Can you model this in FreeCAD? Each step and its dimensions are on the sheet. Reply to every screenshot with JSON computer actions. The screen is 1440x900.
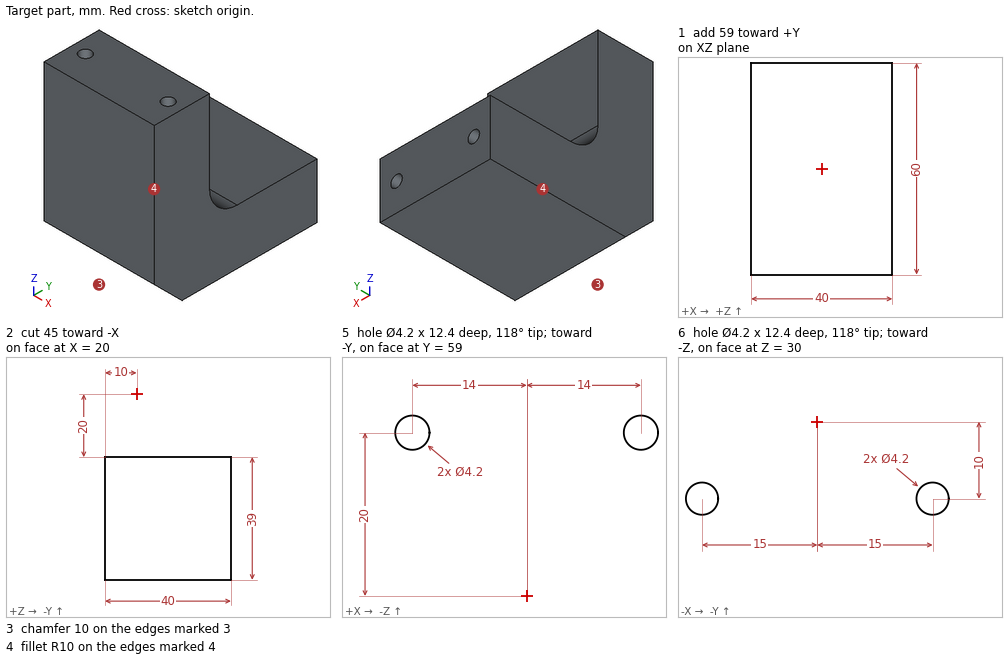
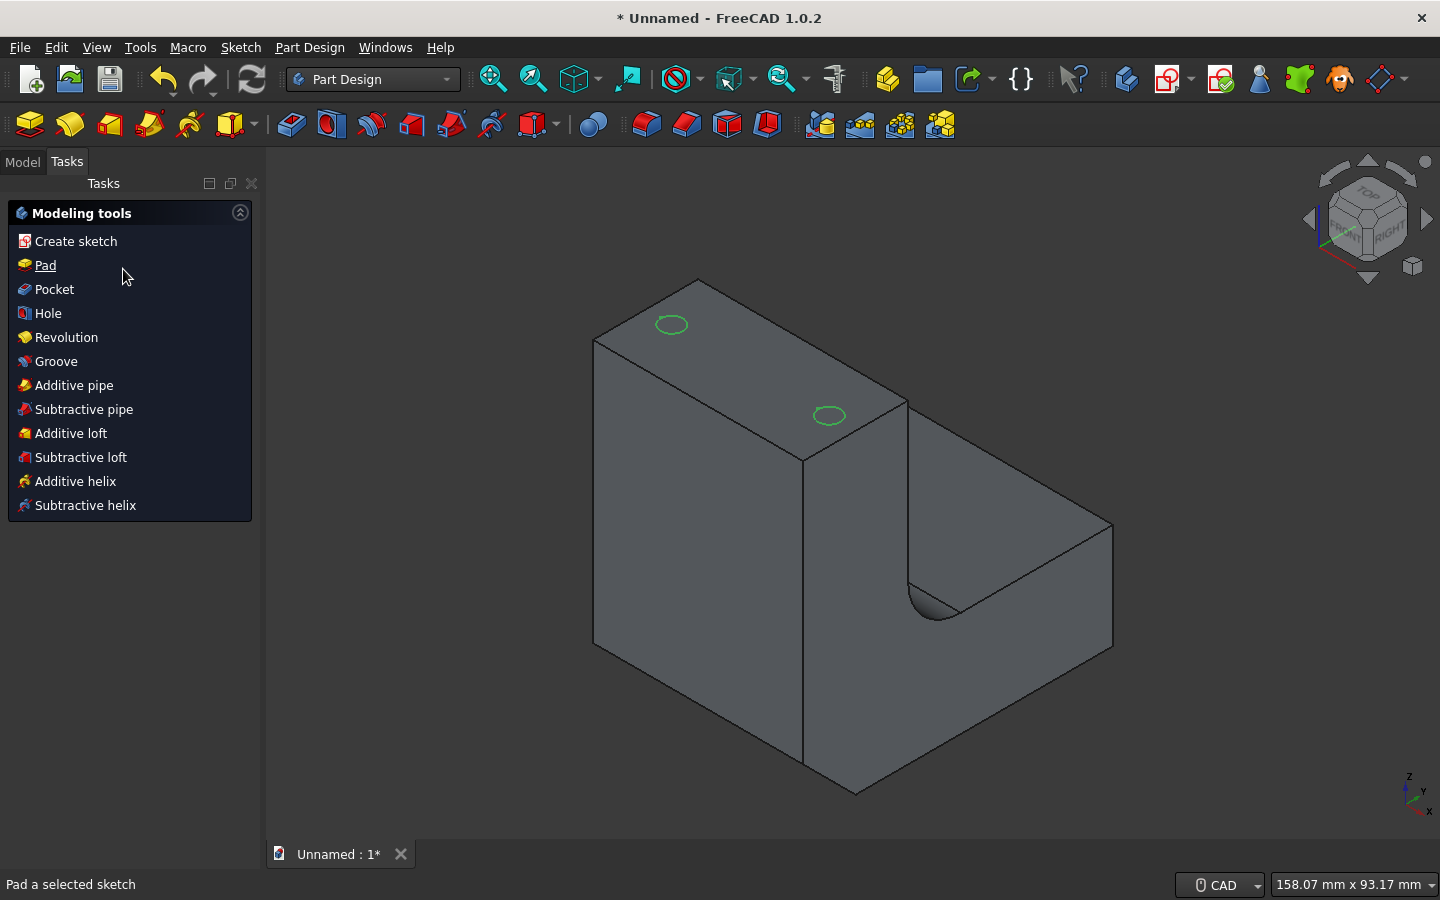
{"action": "left_click", "coordinate": [332, 124]}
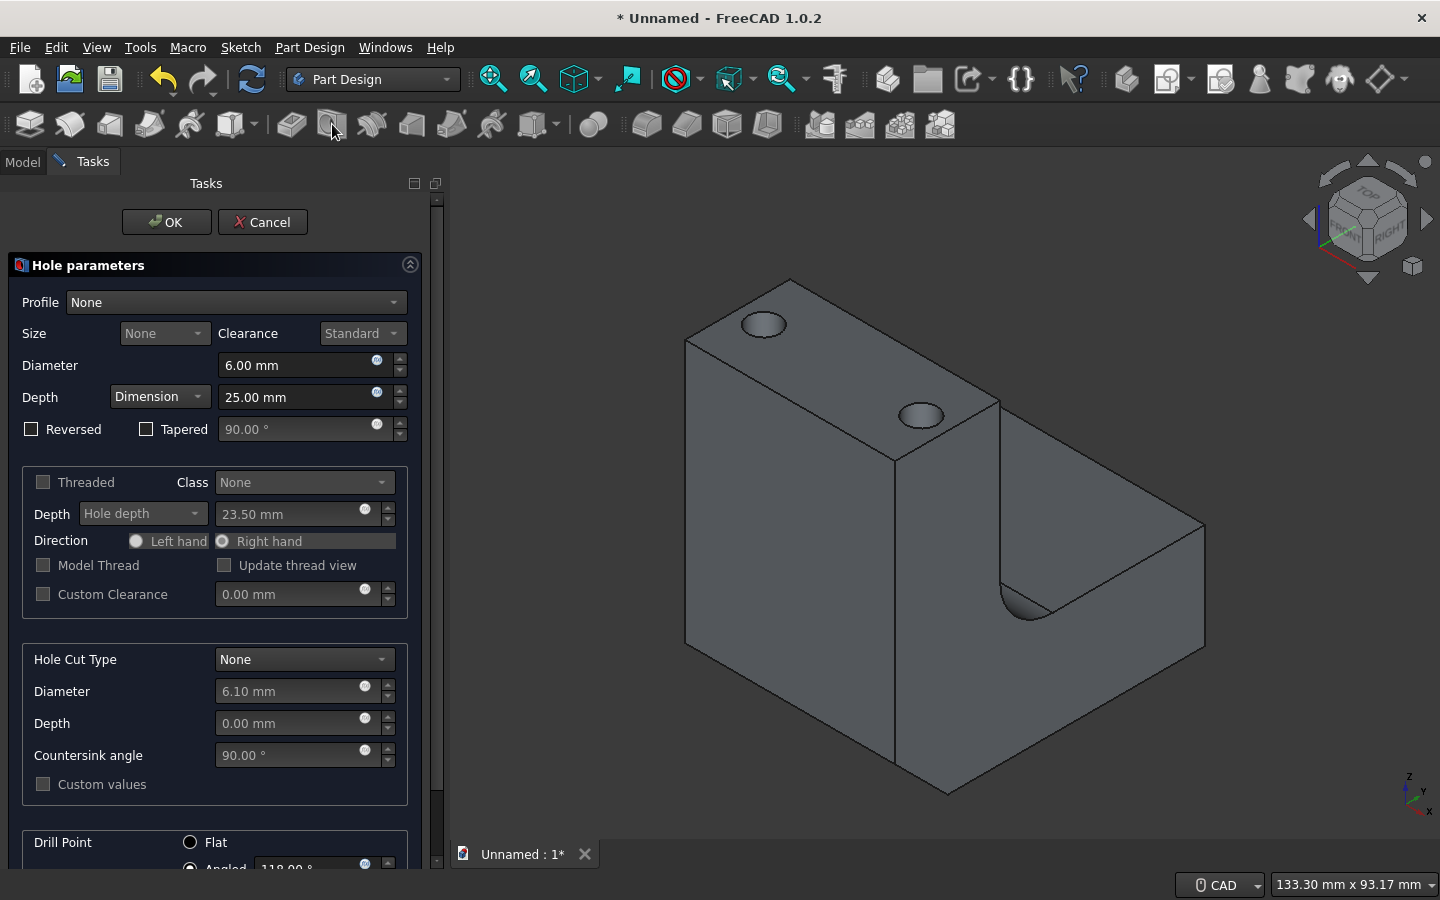
{"action": "triple_click", "coordinate": [305, 365]}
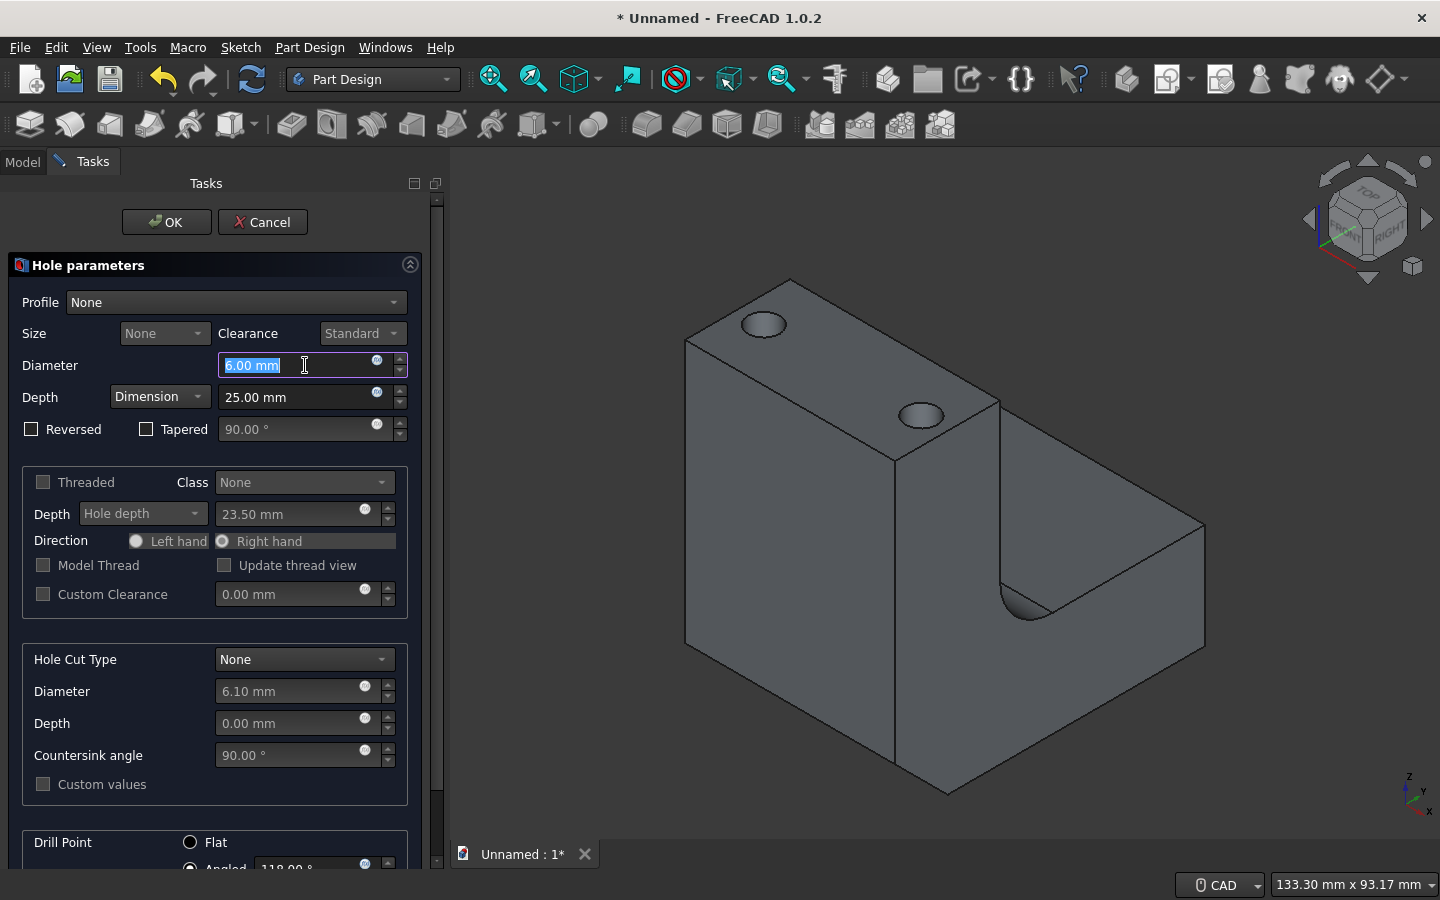
{"action": "type", "text": "4.2"}
{"action": "key", "text": "Tab"}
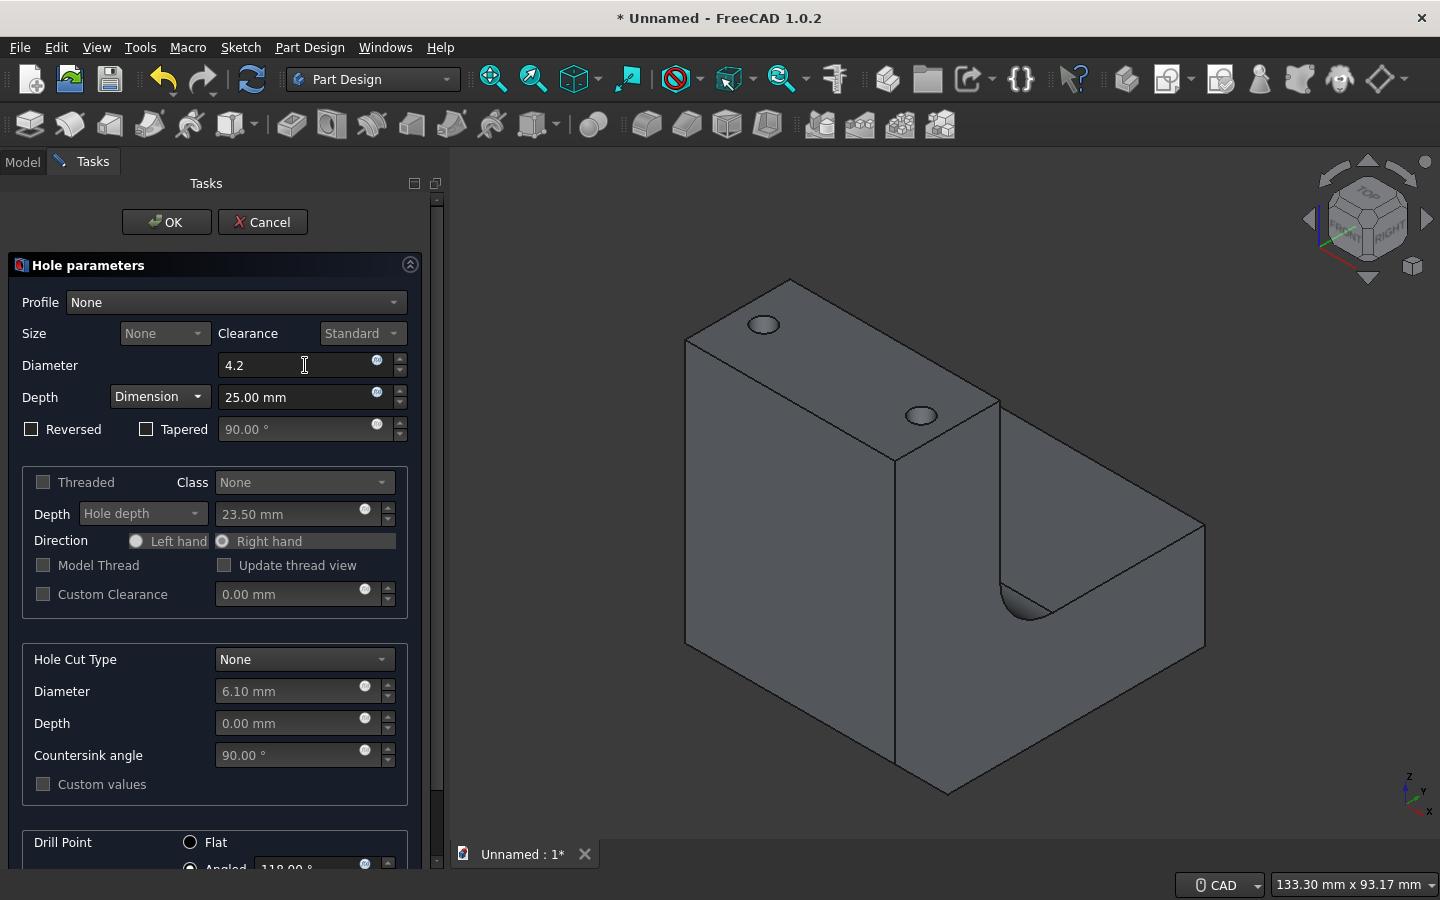
{"action": "triple_click", "coordinate": [305, 397]}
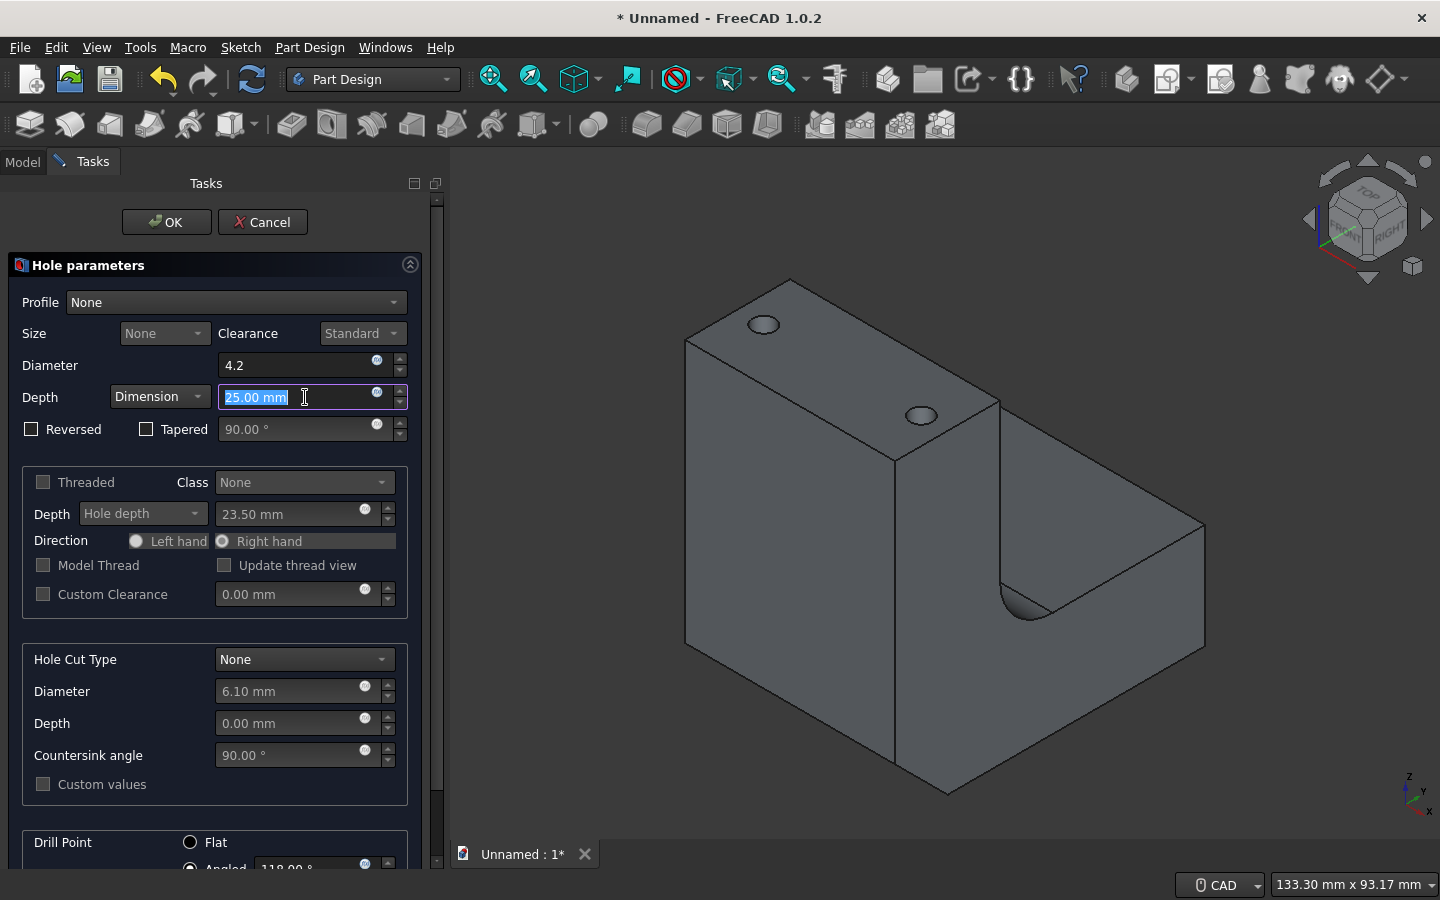
{"action": "type", "text": "12.4"}
{"action": "key", "text": "Tab"}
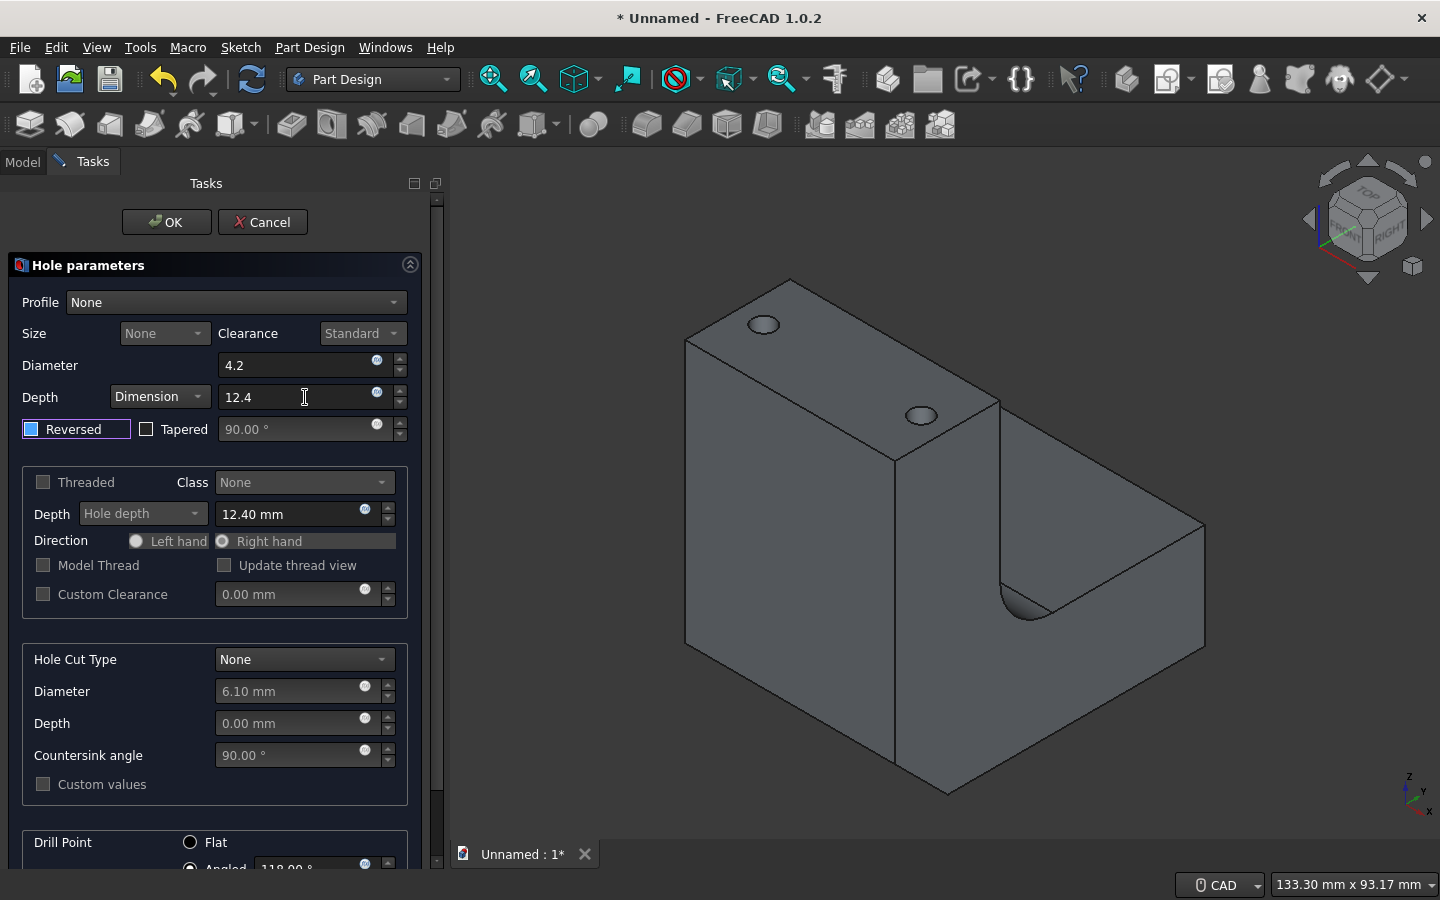
{"action": "left_click", "coordinate": [167, 222]}